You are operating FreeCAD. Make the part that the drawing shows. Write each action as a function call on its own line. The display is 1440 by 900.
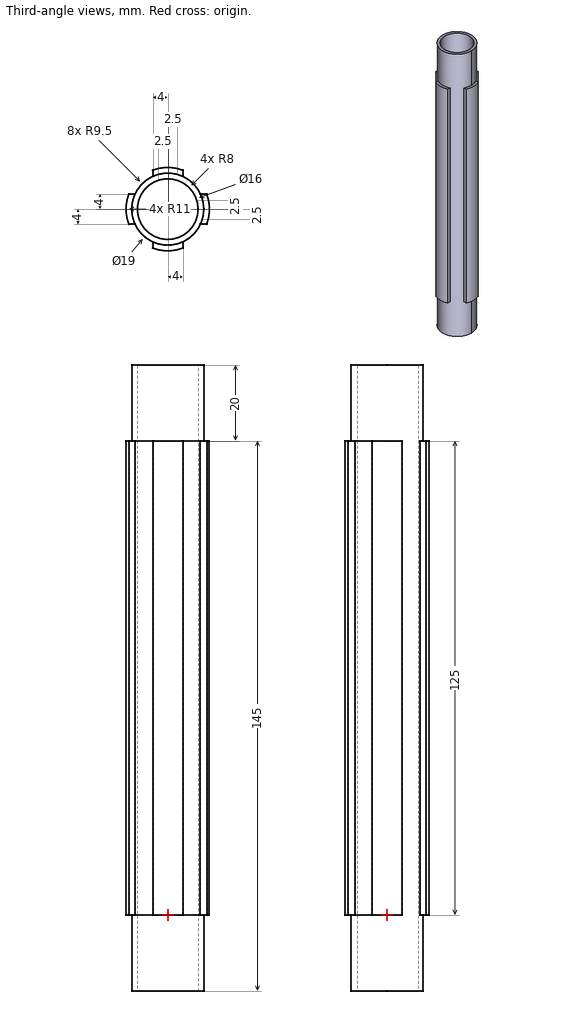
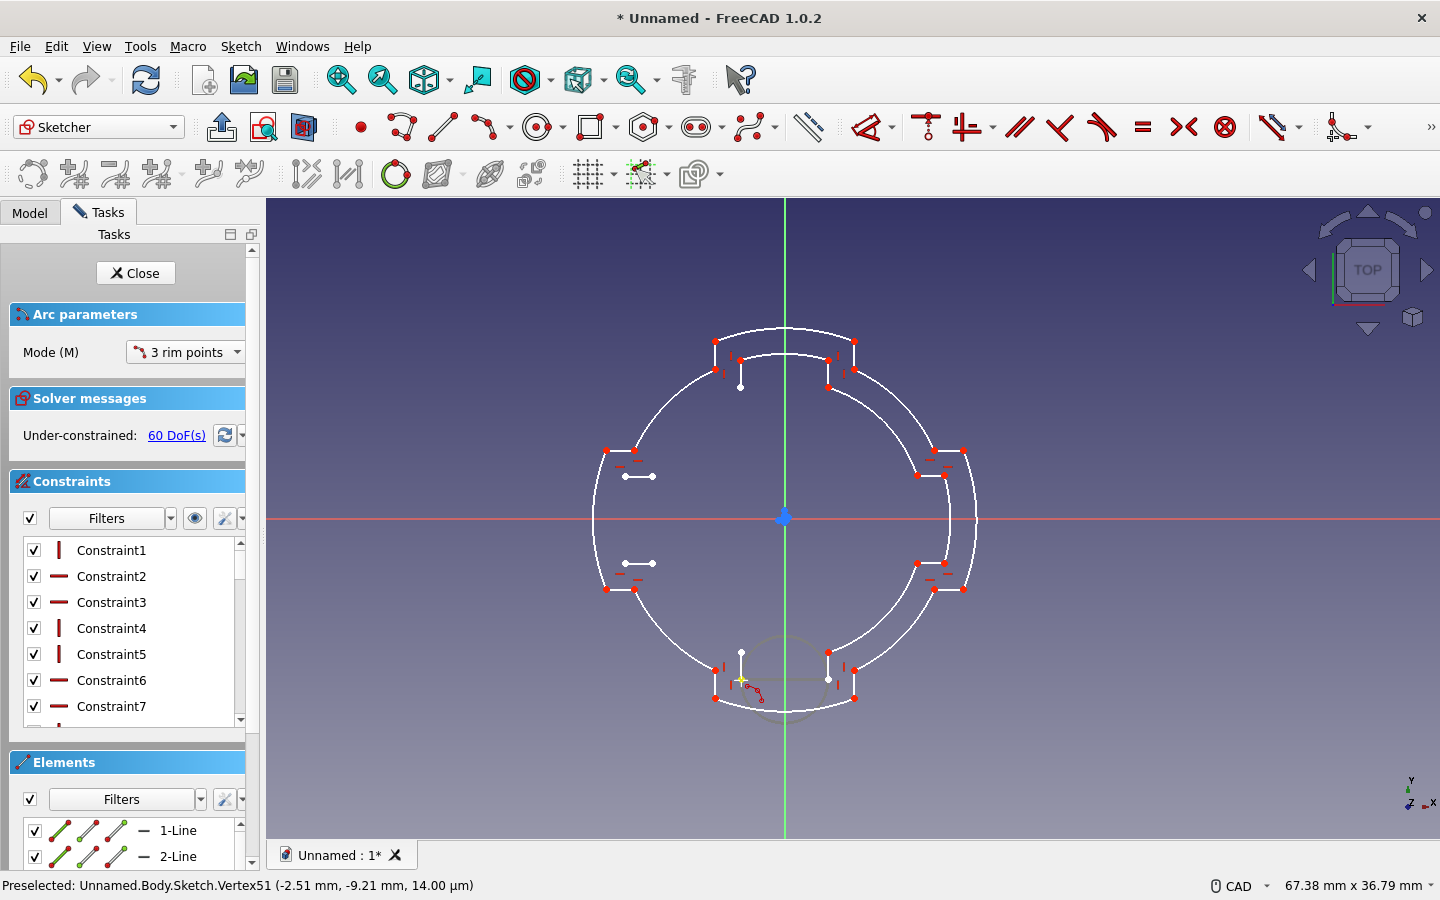
scroll(794, 684, up, 6)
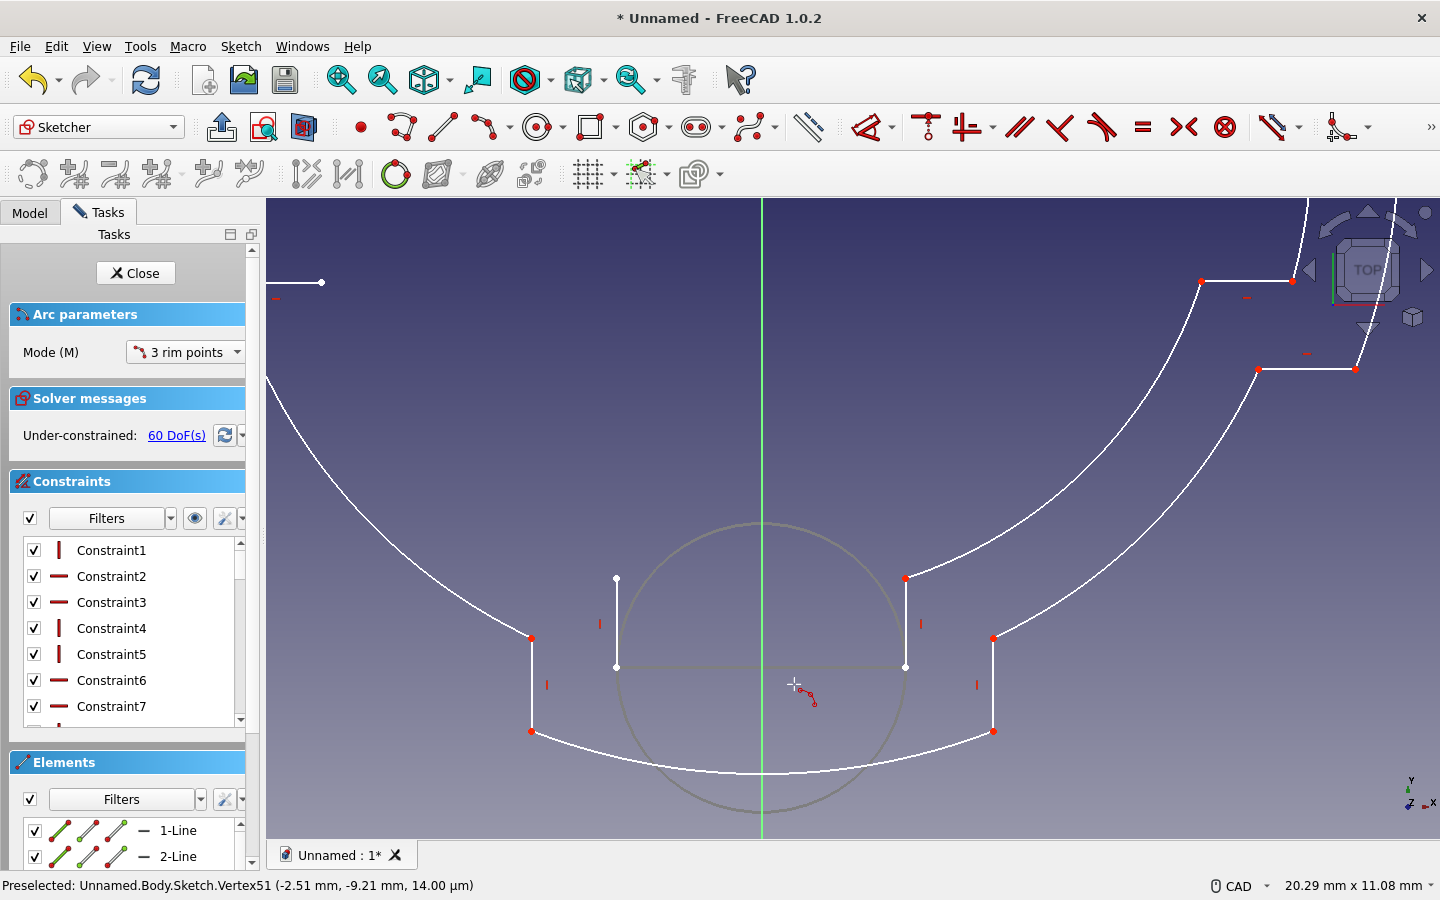
click(791, 684)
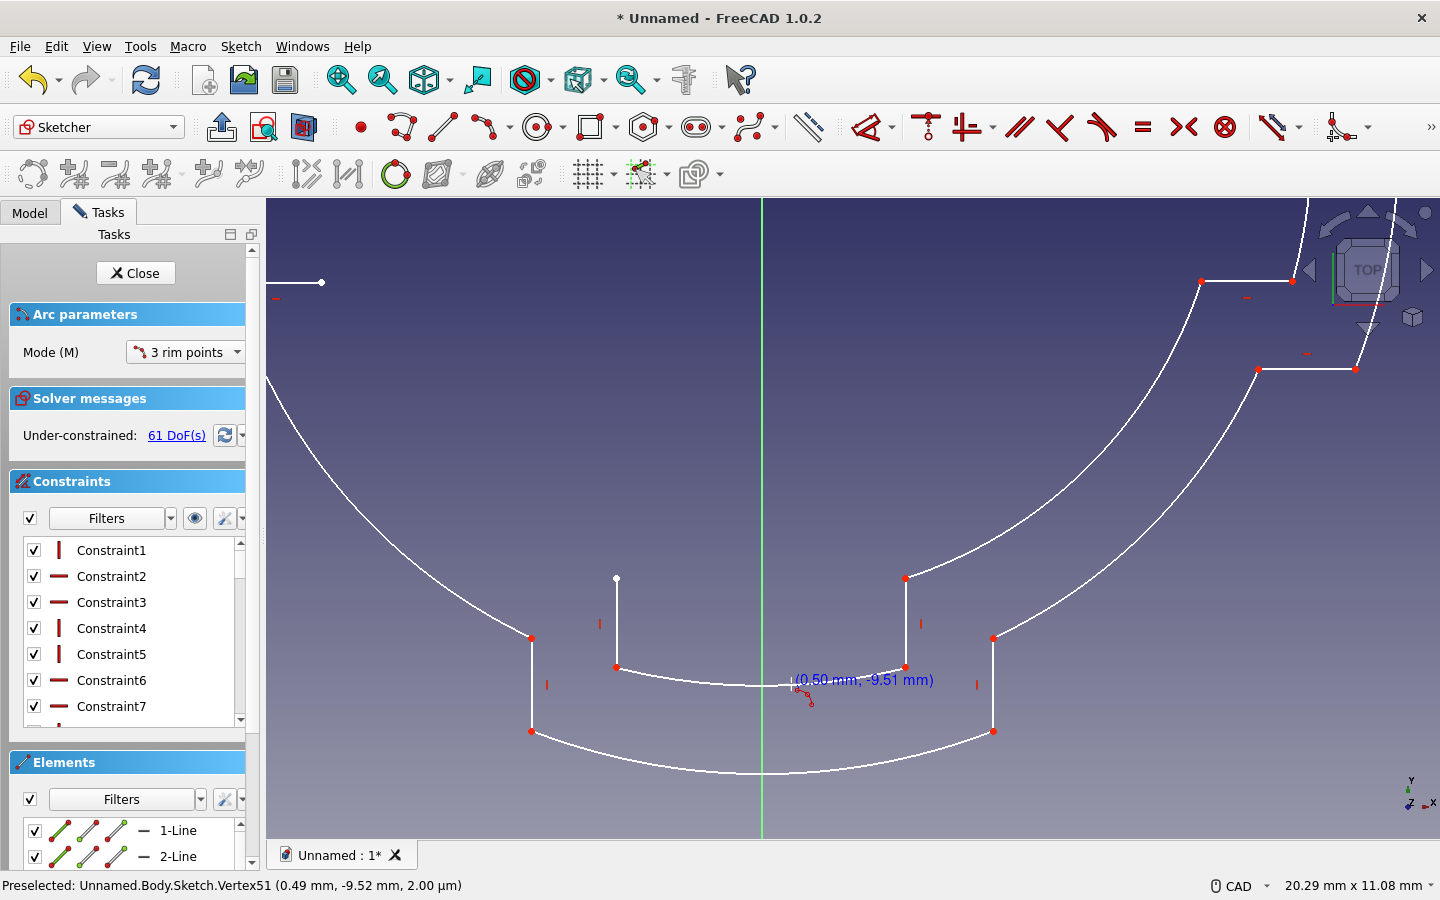
click(617, 578)
click(321, 283)
click(435, 462)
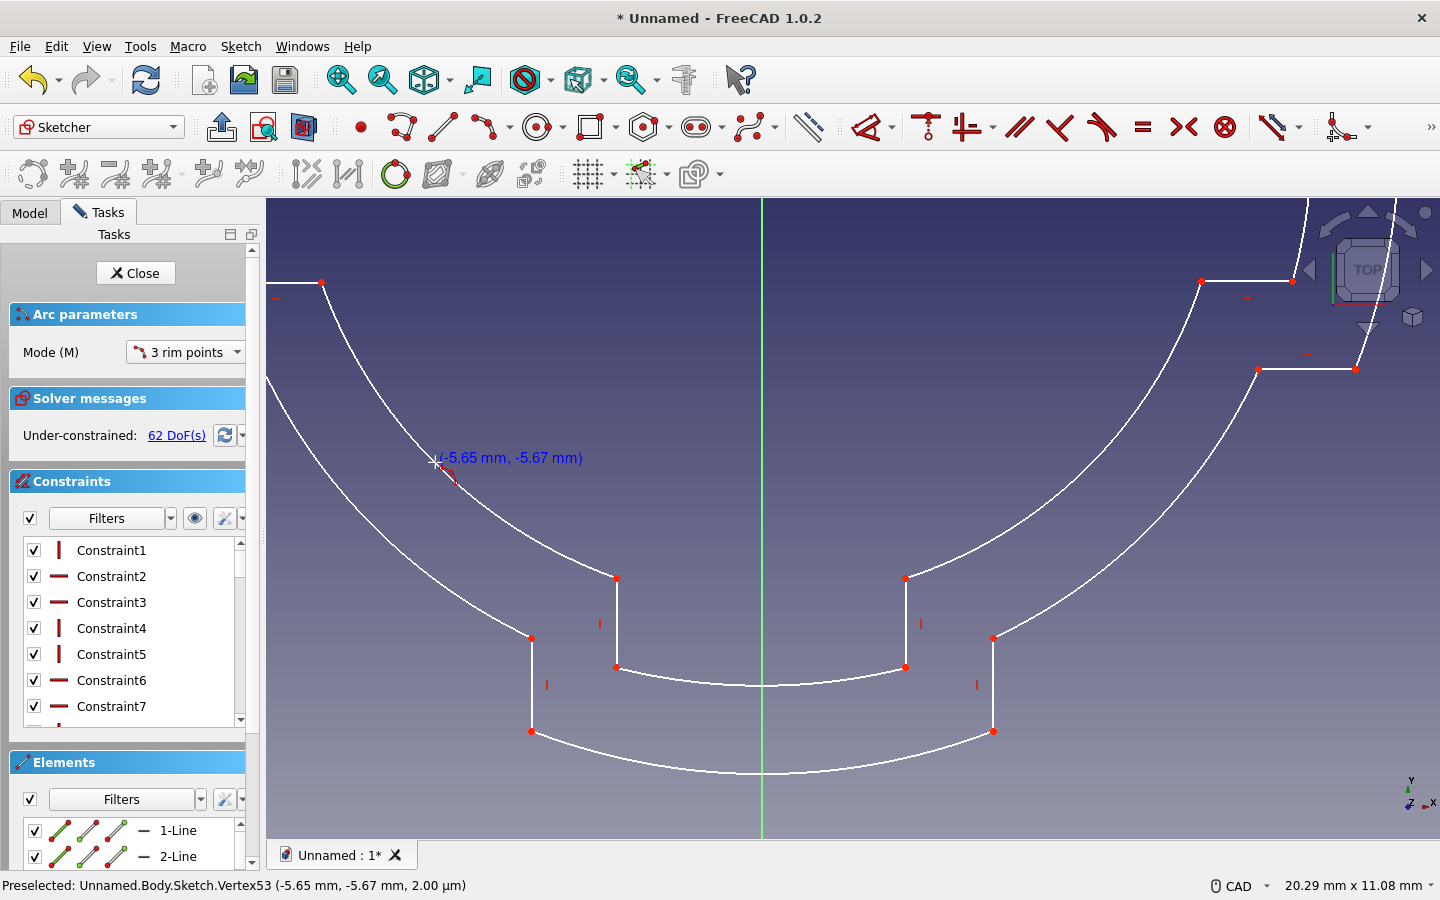
scroll(794, 684, down, 6)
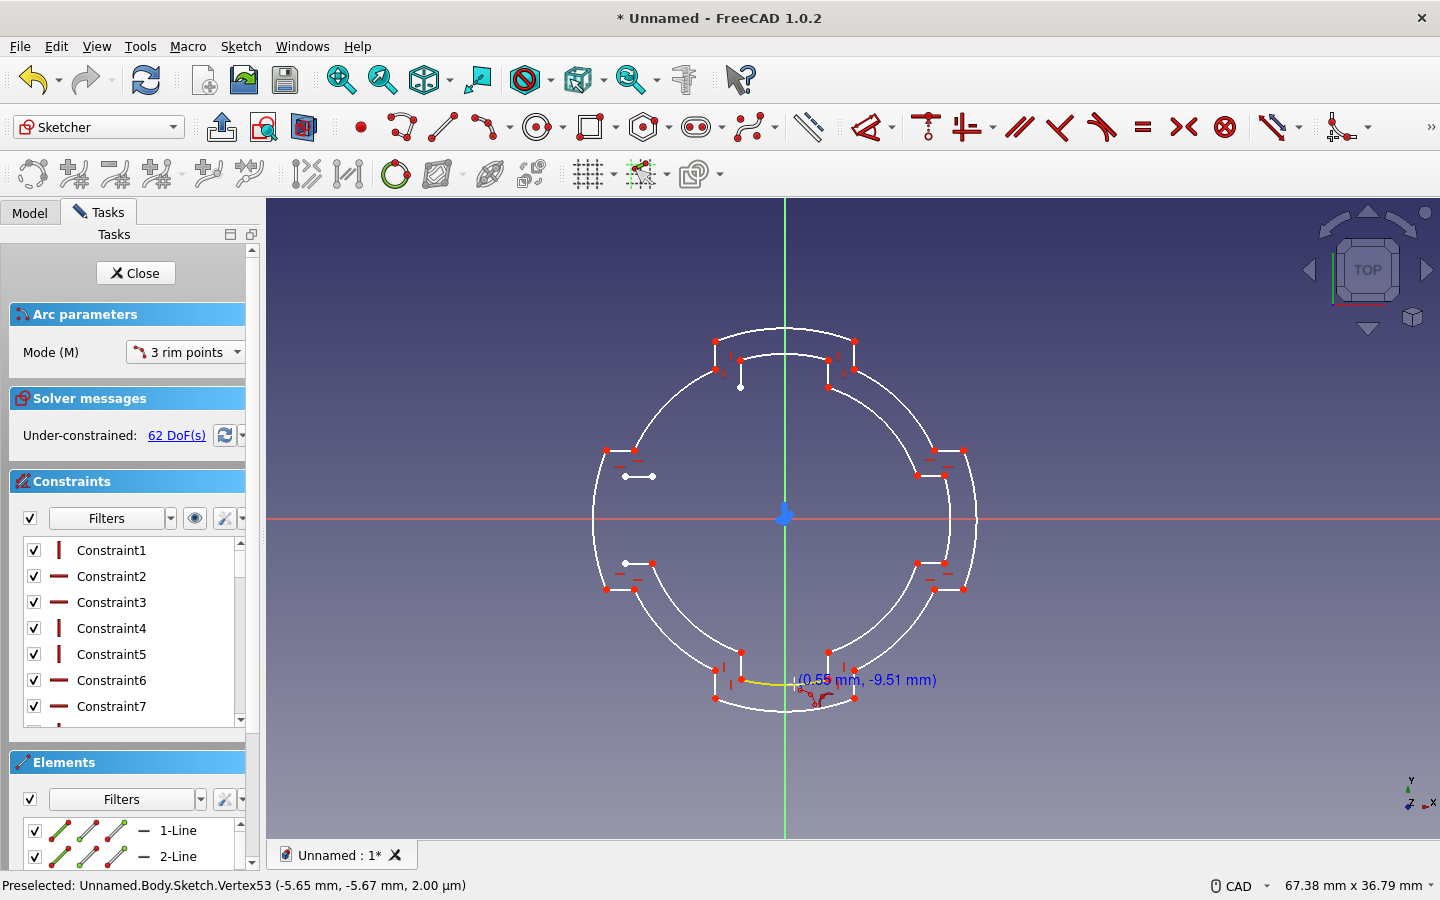
click(625, 564)
click(625, 477)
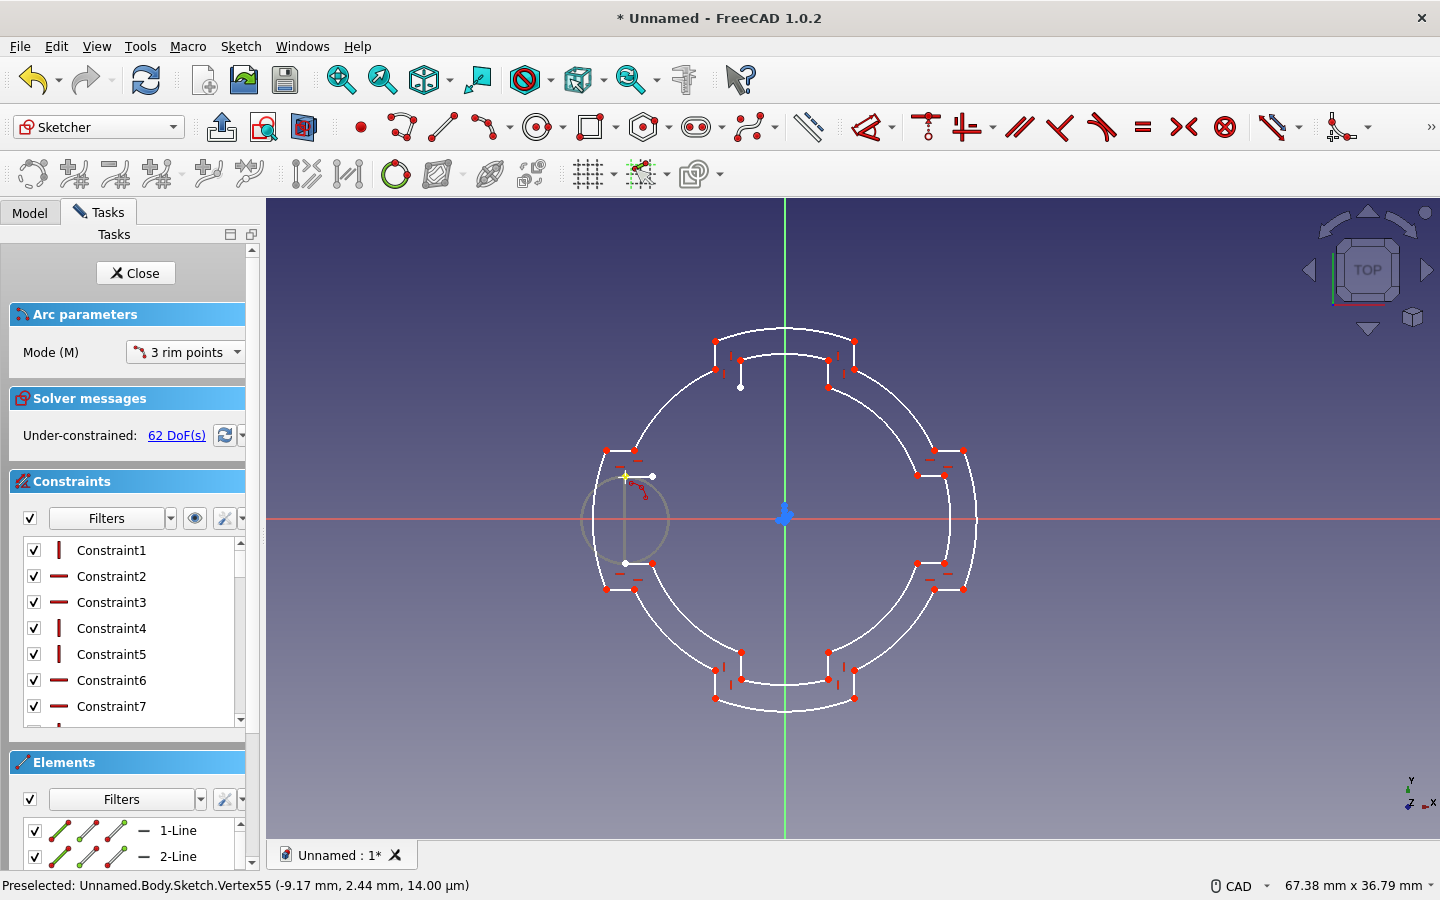
scroll(619, 528, up, 6)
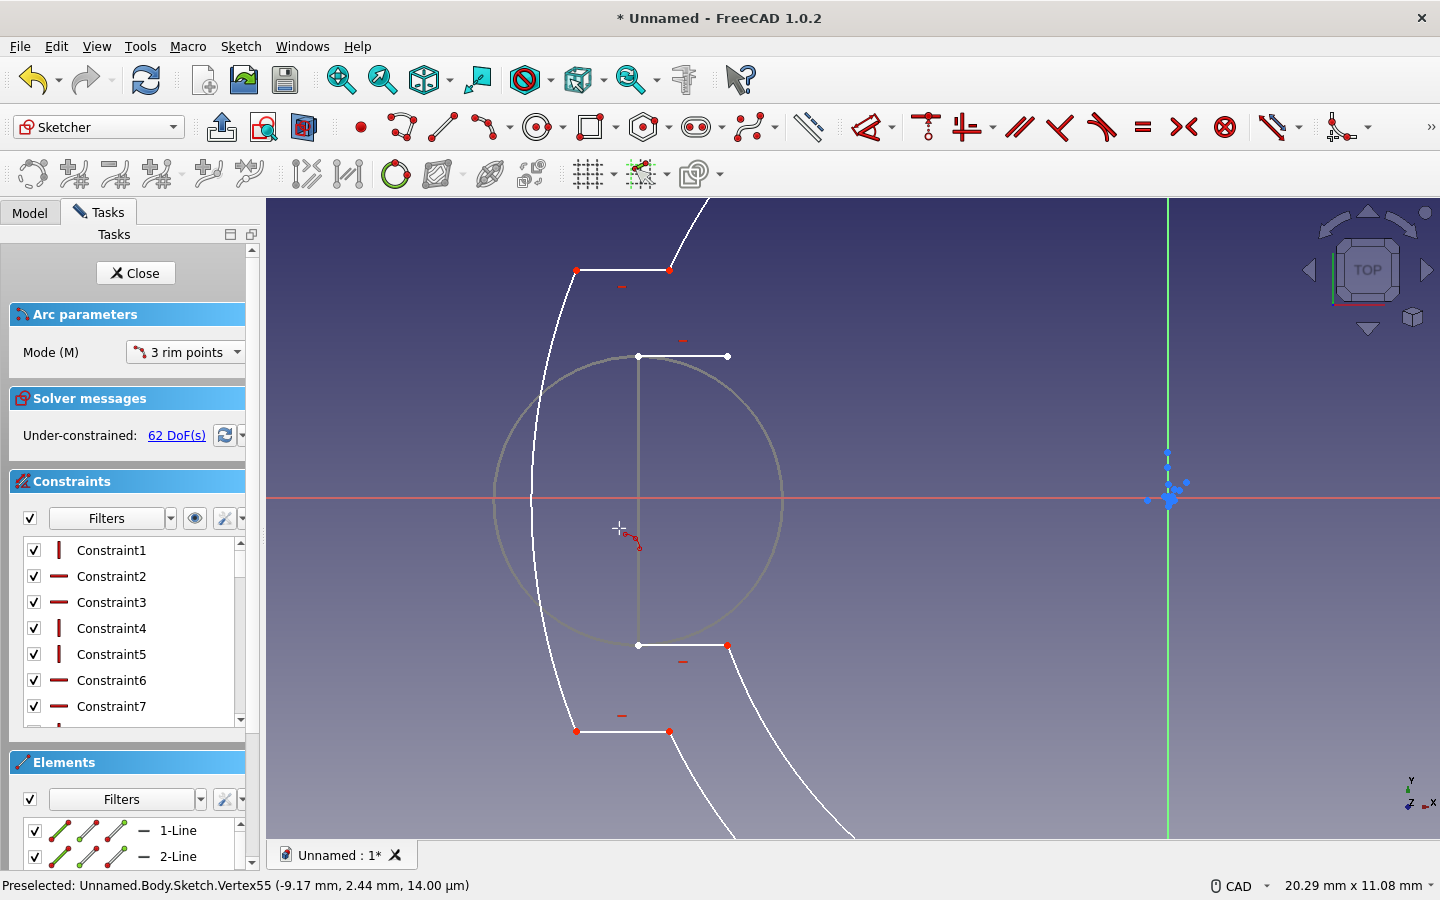
click(620, 527)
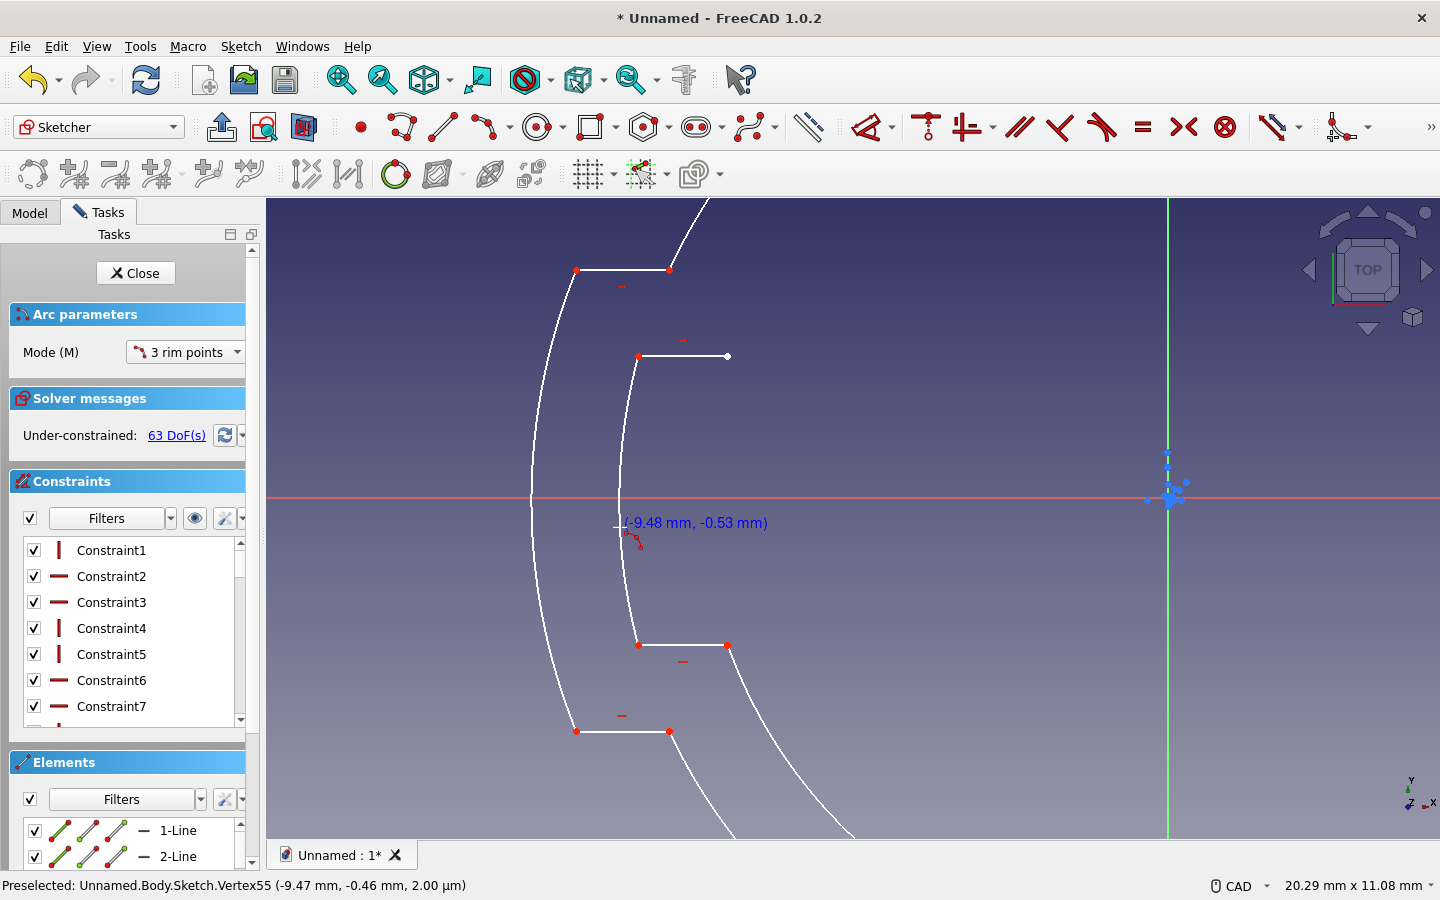
click(728, 356)